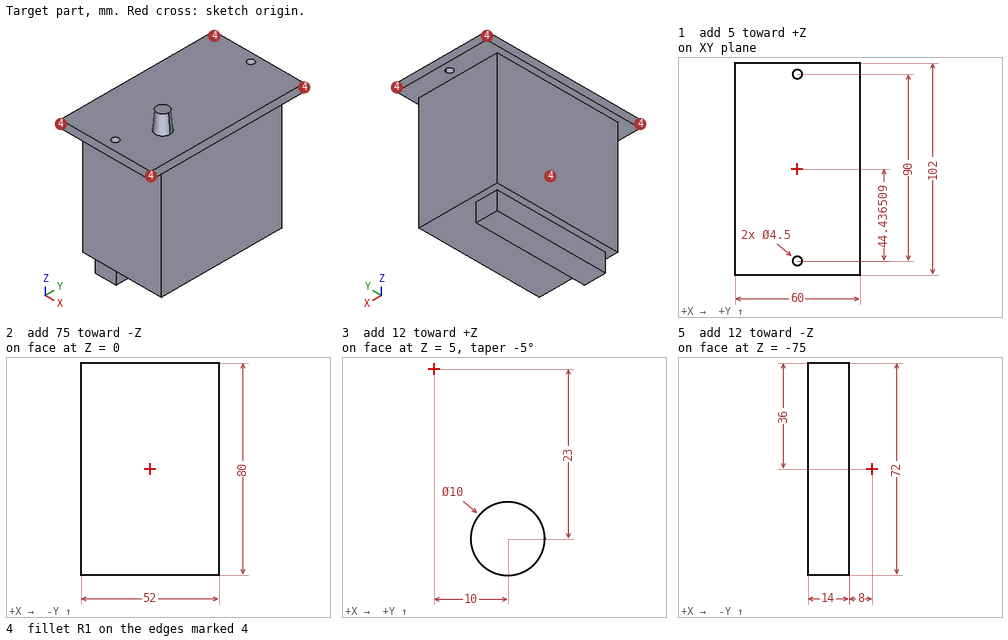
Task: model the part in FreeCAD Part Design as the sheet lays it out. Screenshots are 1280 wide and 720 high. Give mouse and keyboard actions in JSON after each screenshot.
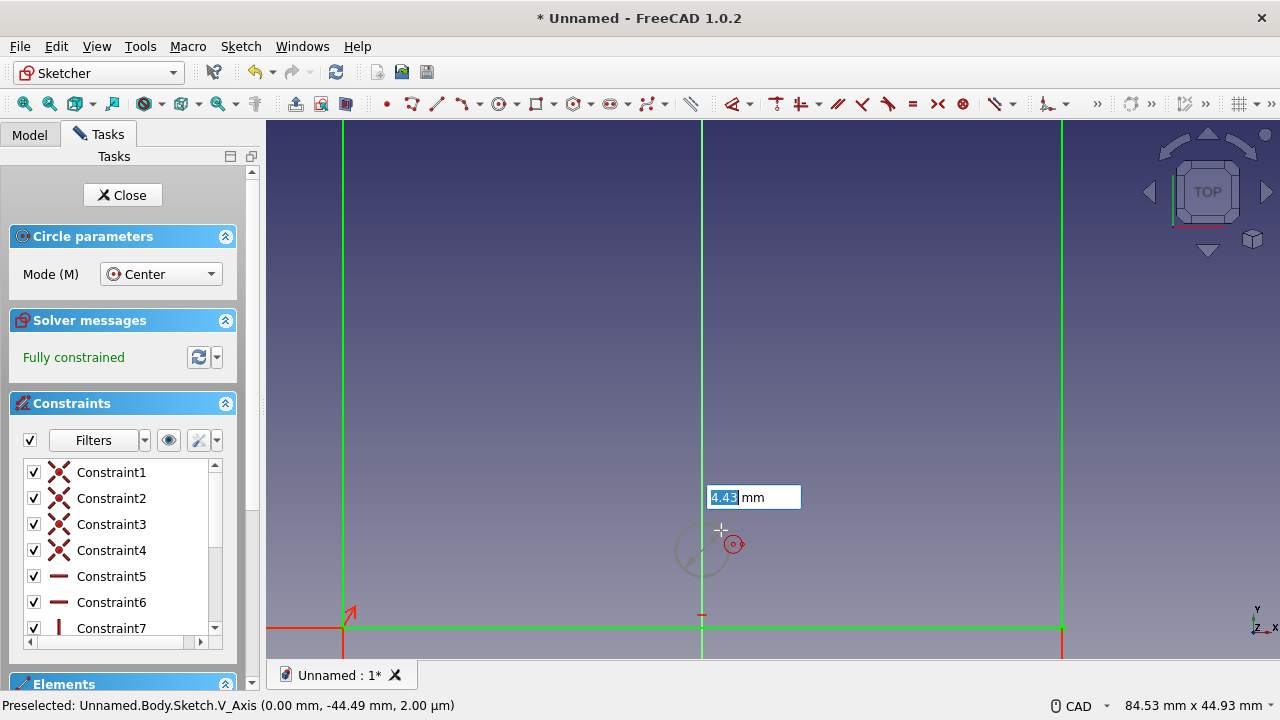
{"action": "type", "text": "4.5"}
{"action": "key", "text": "Return"}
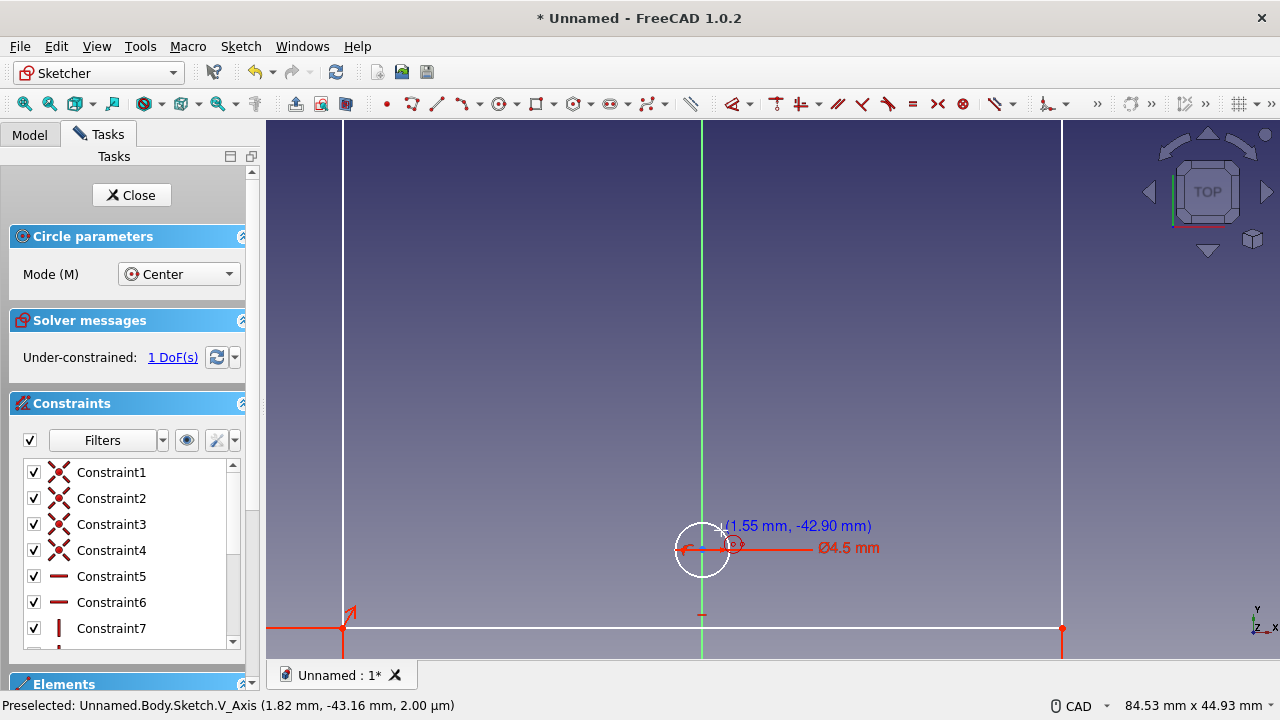
{"action": "scroll", "coordinate": [705, 550], "scroll_direction": "down", "scroll_amount": 6}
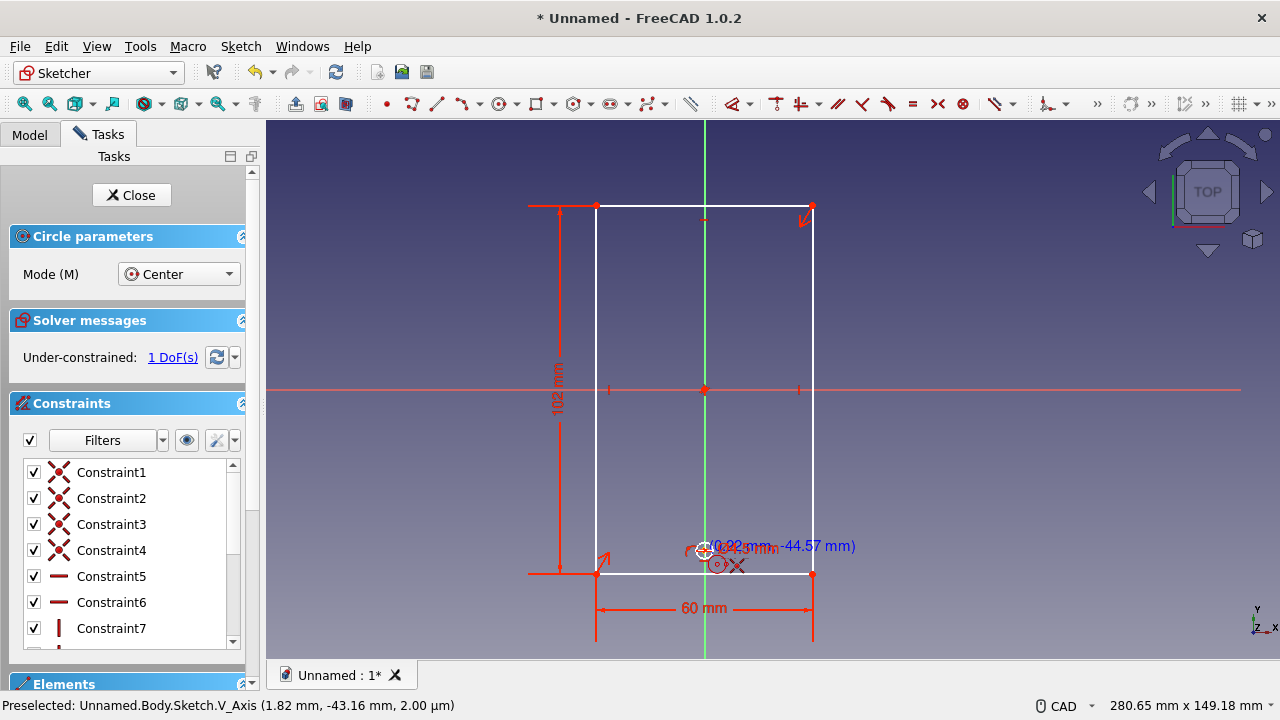
{"action": "scroll", "coordinate": [705, 225], "scroll_direction": "up", "scroll_amount": 6}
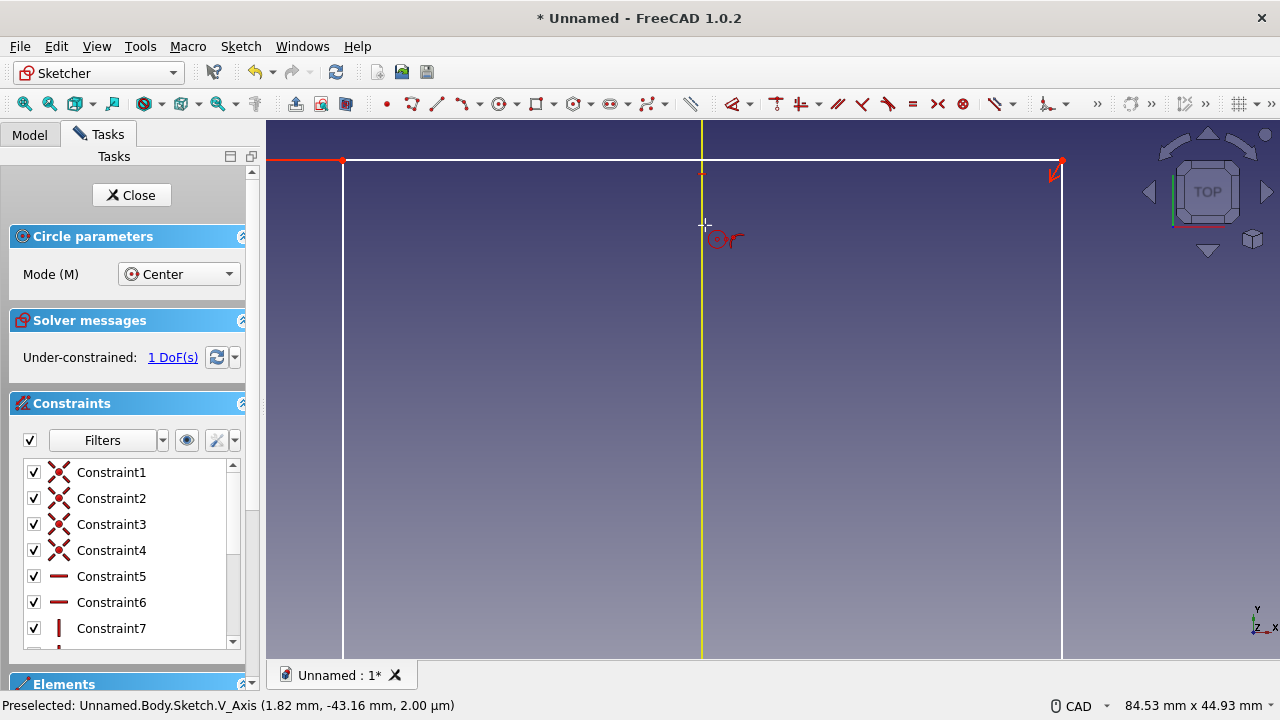
{"action": "left_click", "coordinate": [702, 225]}
{"action": "mouse_move", "coordinate": [721, 206]}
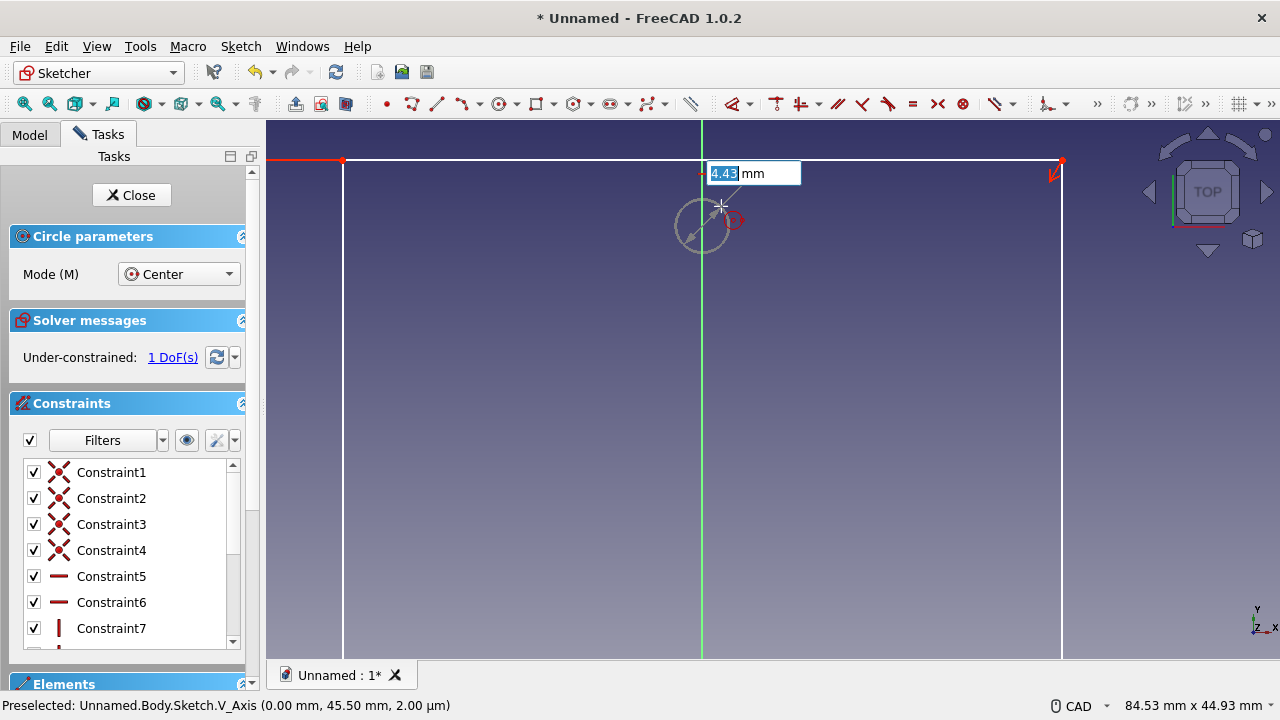
{"action": "type", "text": "4.5"}
{"action": "key", "text": "Return"}
{"action": "key", "text": "Escape"}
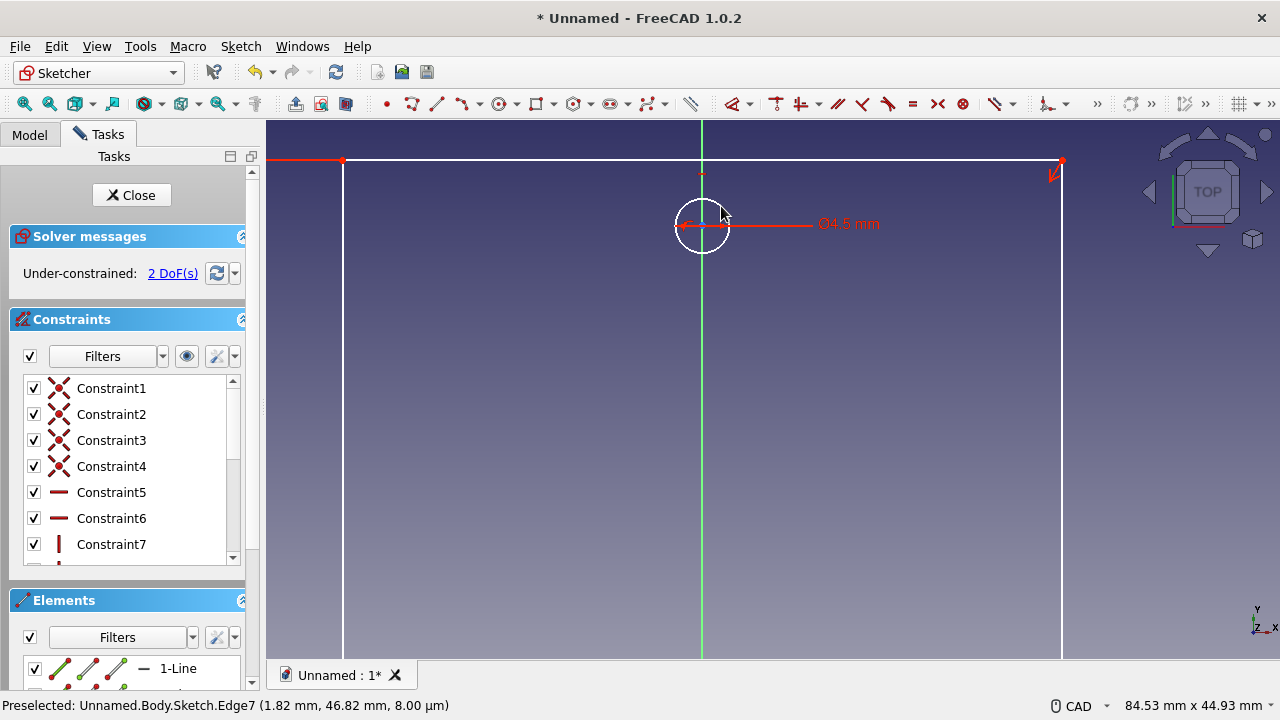
{"action": "key", "text": "d"}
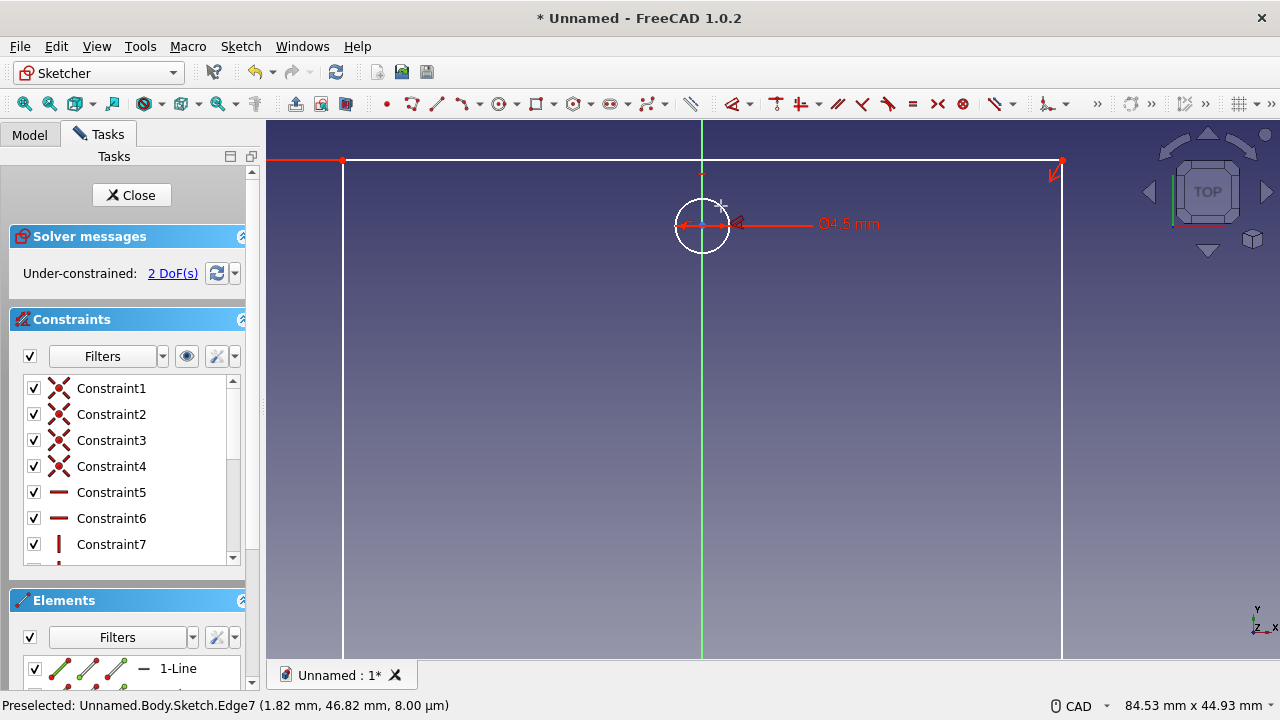
{"action": "scroll", "coordinate": [705, 225], "scroll_direction": "down", "scroll_amount": 6}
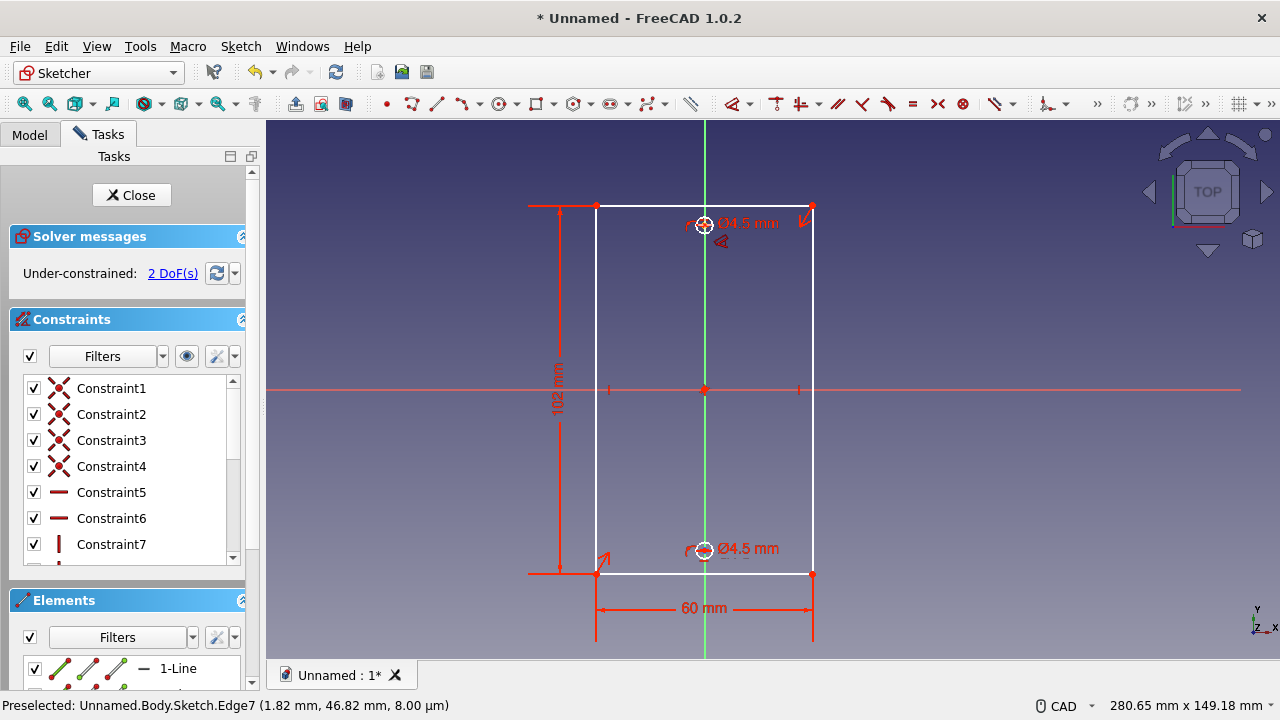
{"action": "left_click", "coordinate": [705, 551]}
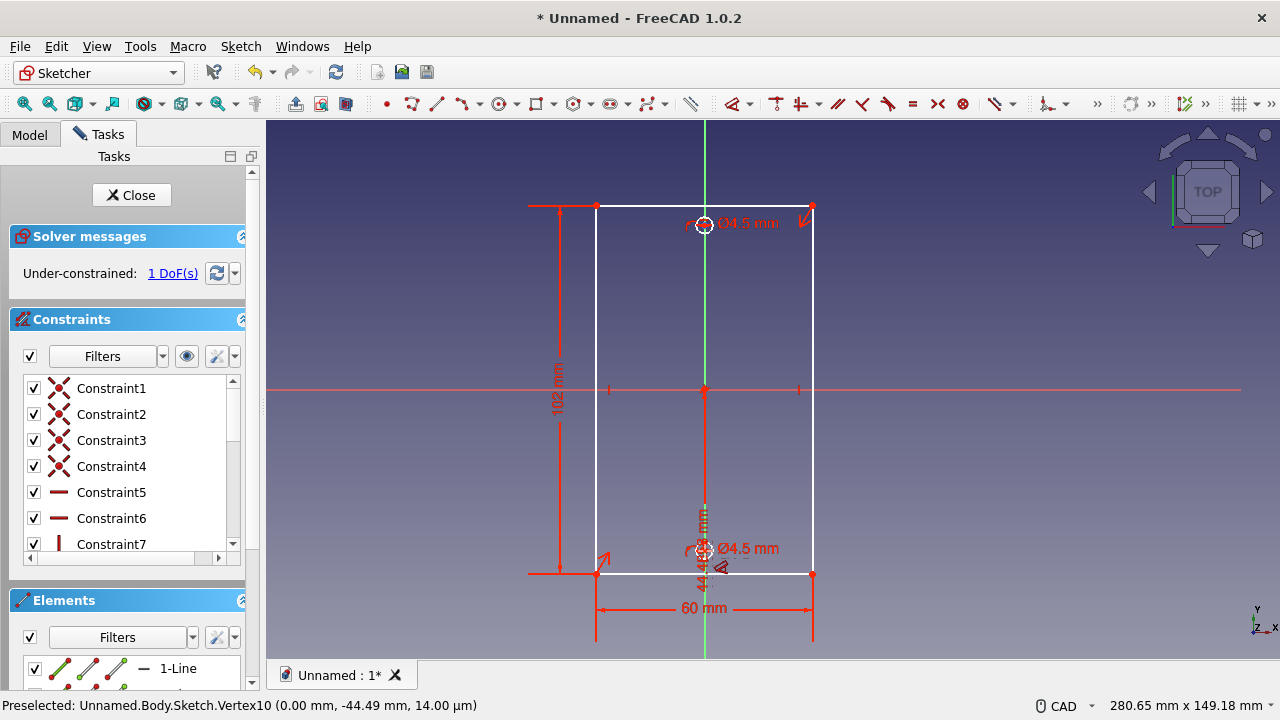
{"action": "left_click", "coordinate": [705, 225]}
{"action": "left_click", "coordinate": [739, 313]}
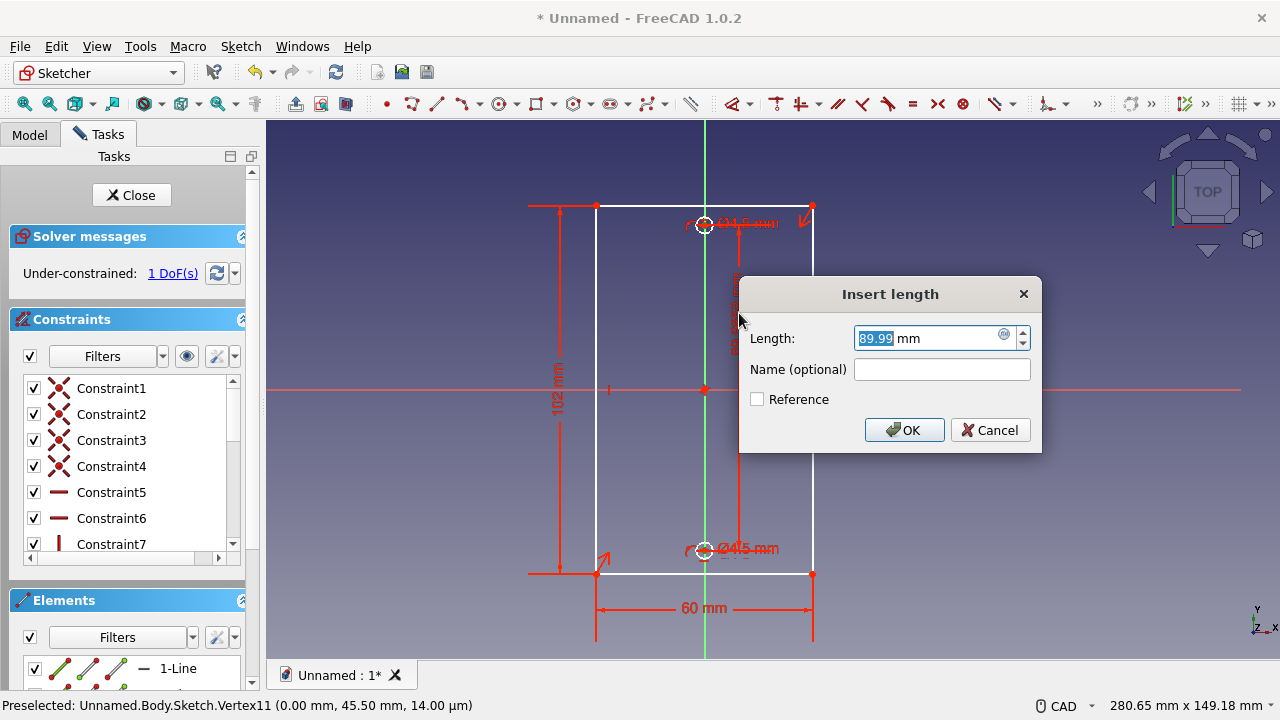
{"action": "type", "text": "90"}
{"action": "key", "text": "Return"}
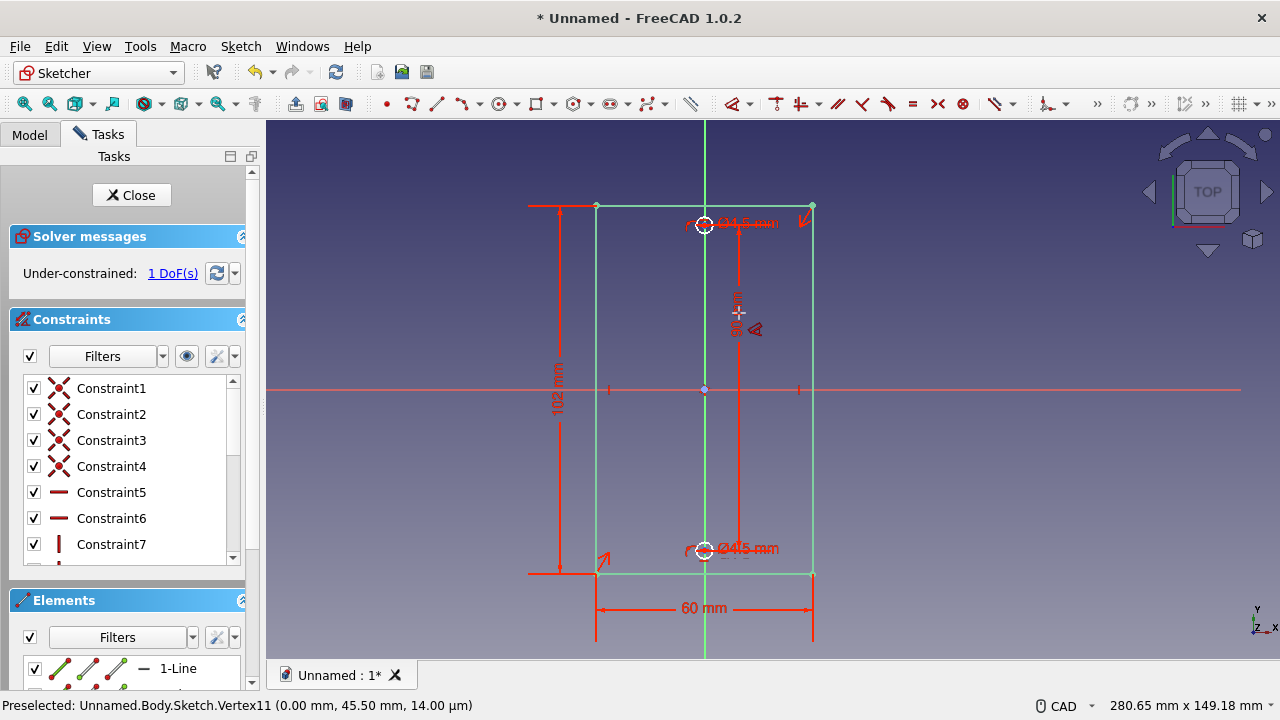
{"action": "left_click", "coordinate": [705, 551]}
{"action": "left_click", "coordinate": [739, 470]}